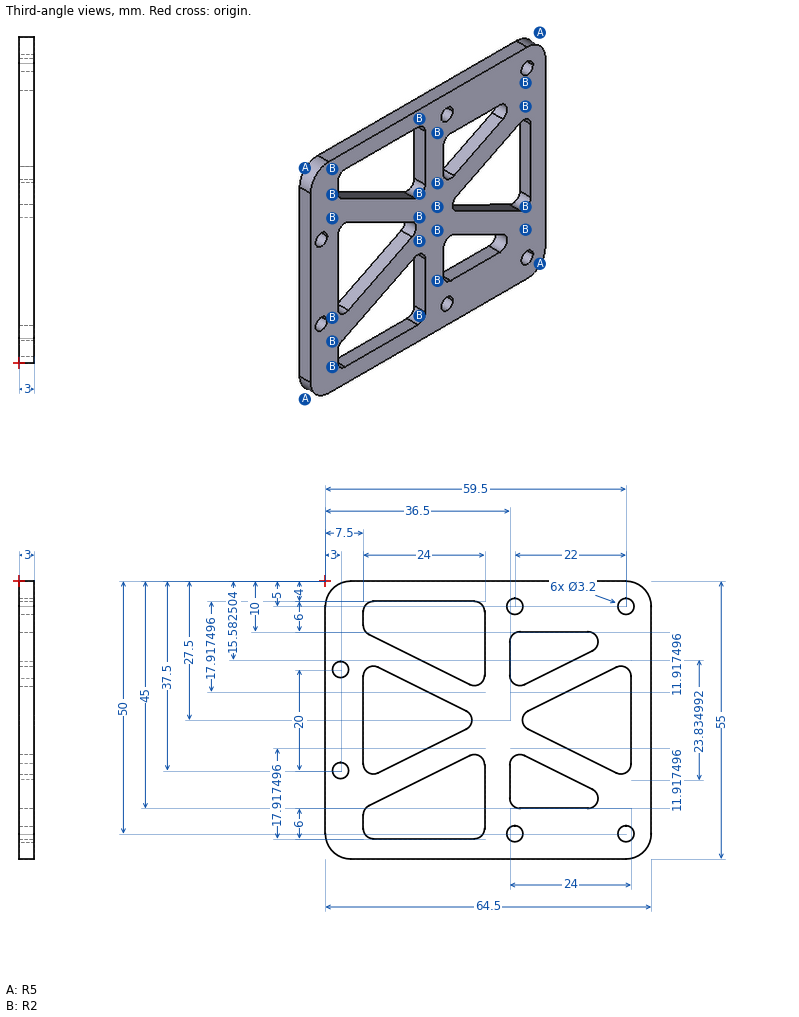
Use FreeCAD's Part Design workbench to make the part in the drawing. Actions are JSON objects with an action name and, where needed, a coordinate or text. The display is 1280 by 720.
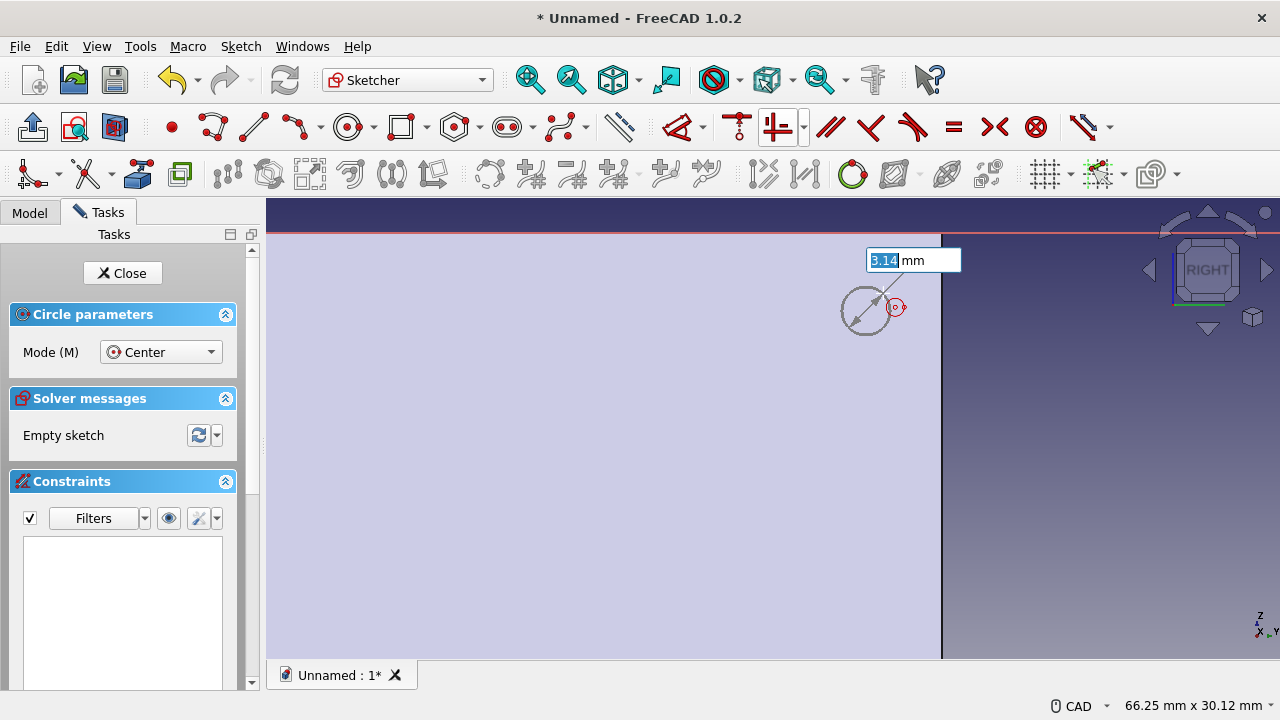
{"action": "type", "text": "3.2"}
{"action": "key", "text": "Return"}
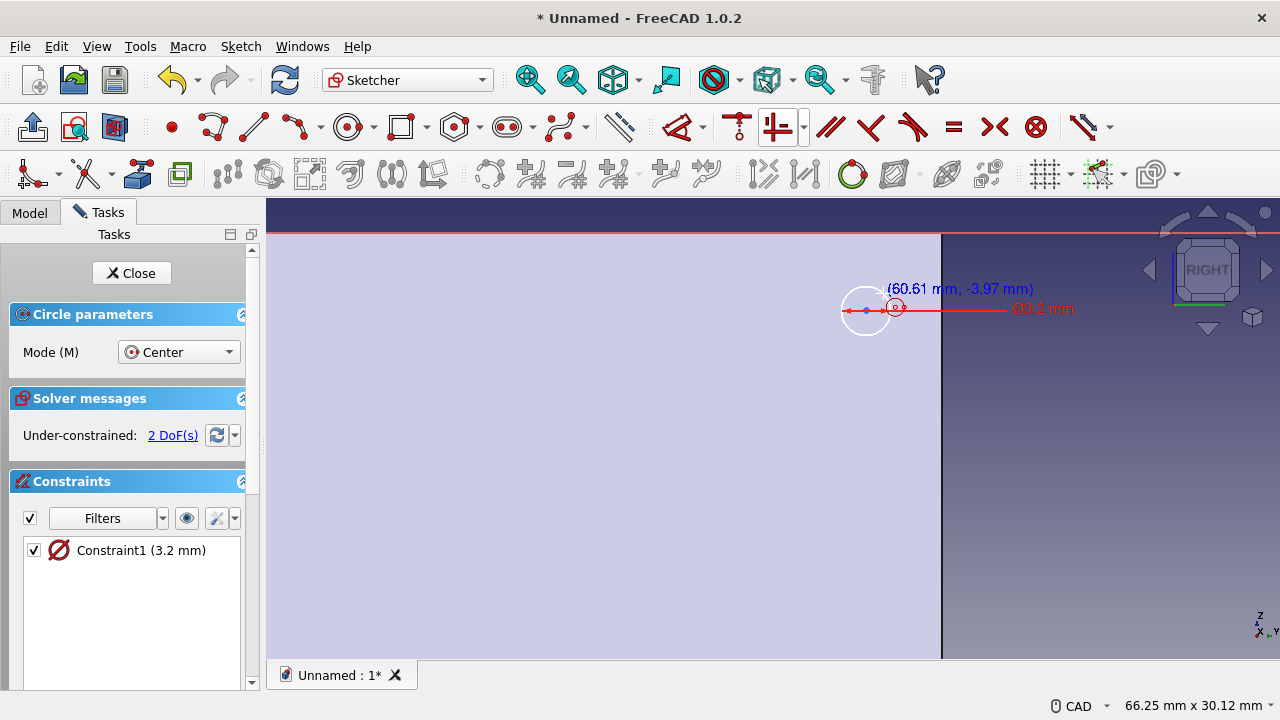
{"action": "left_click", "coordinate": [529, 310]}
{"action": "mouse_move", "coordinate": [547, 293]}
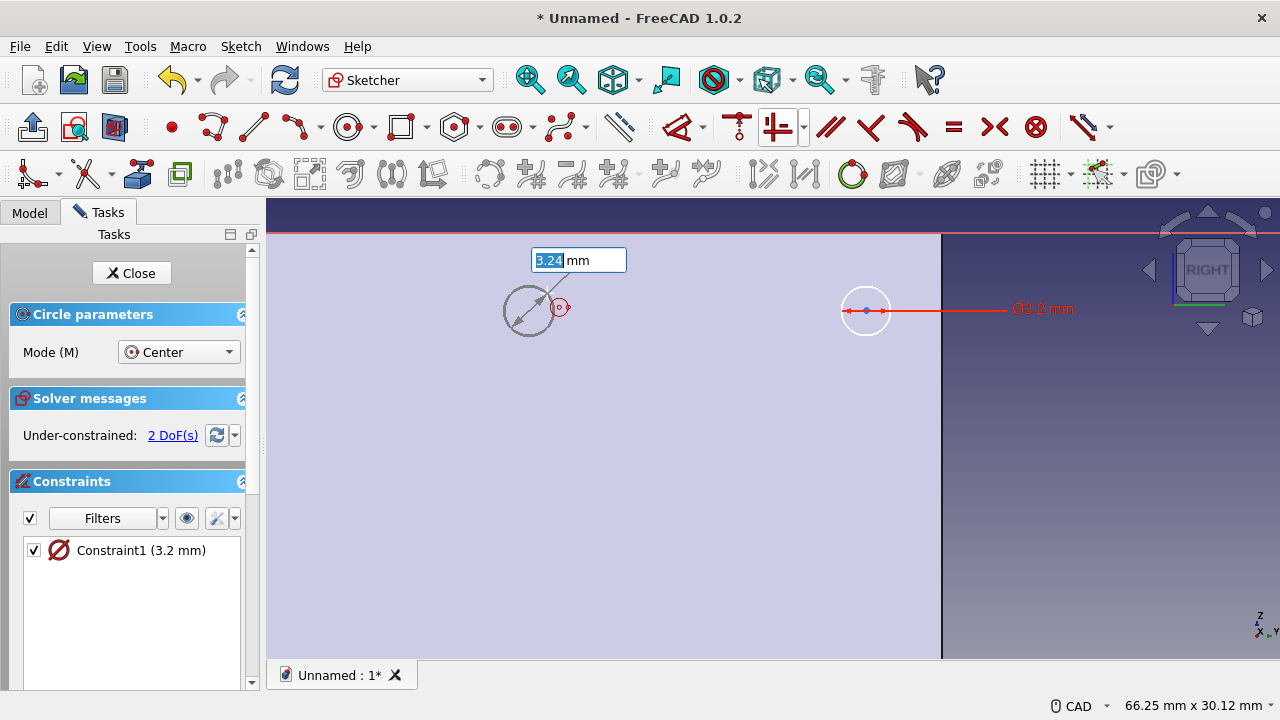
{"action": "type", "text": "3.2"}
{"action": "key", "text": "Return"}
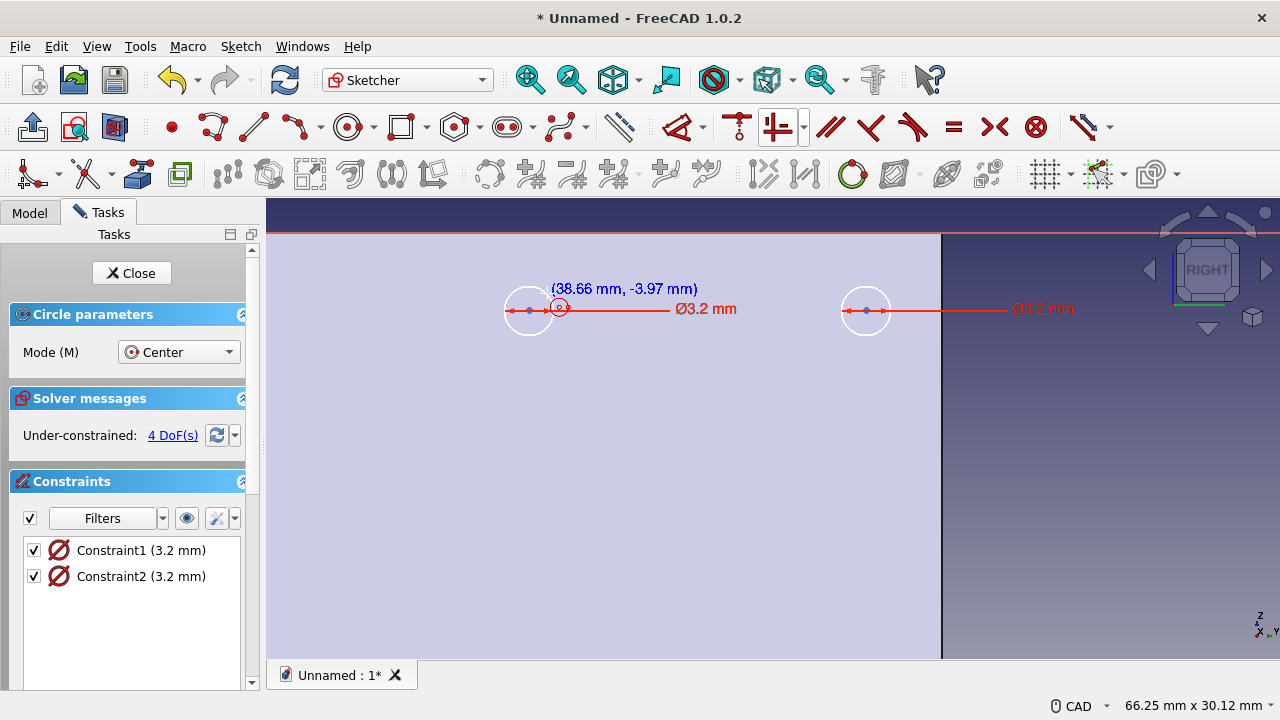
{"action": "scroll", "coordinate": [868, 312], "scroll_direction": "down", "scroll_amount": 5}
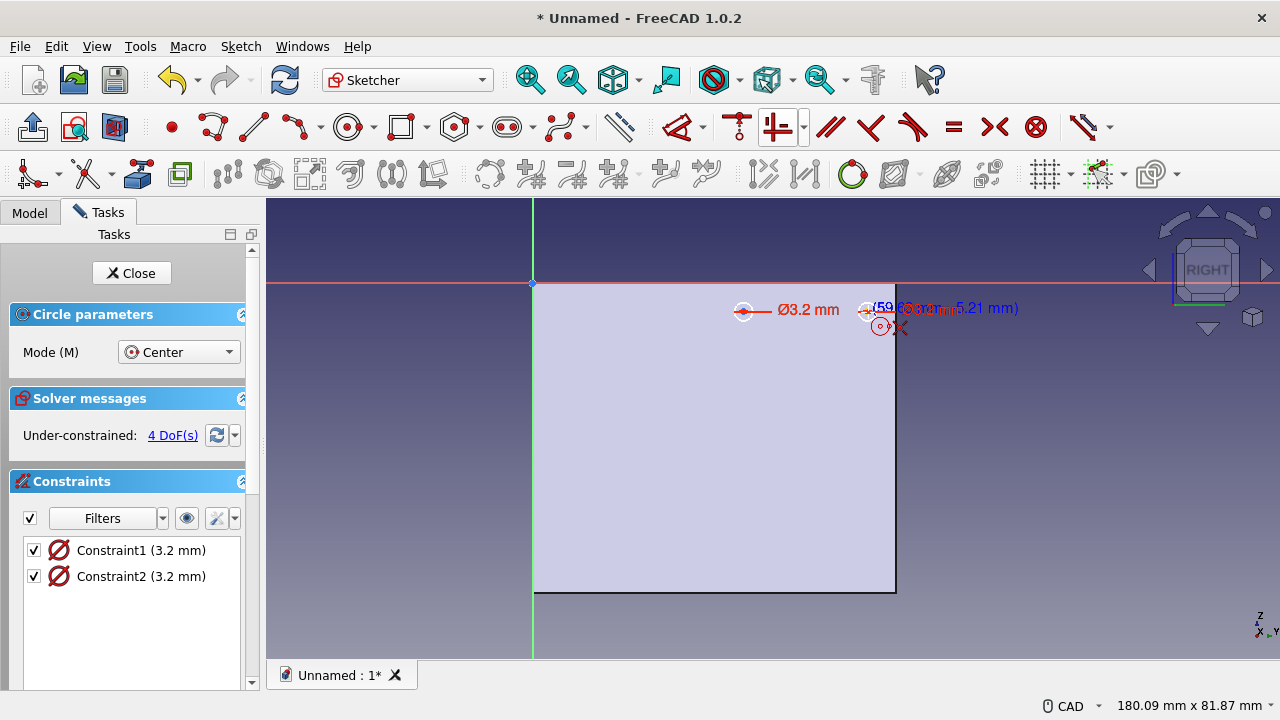
{"action": "scroll", "coordinate": [868, 565], "scroll_direction": "up", "scroll_amount": 5}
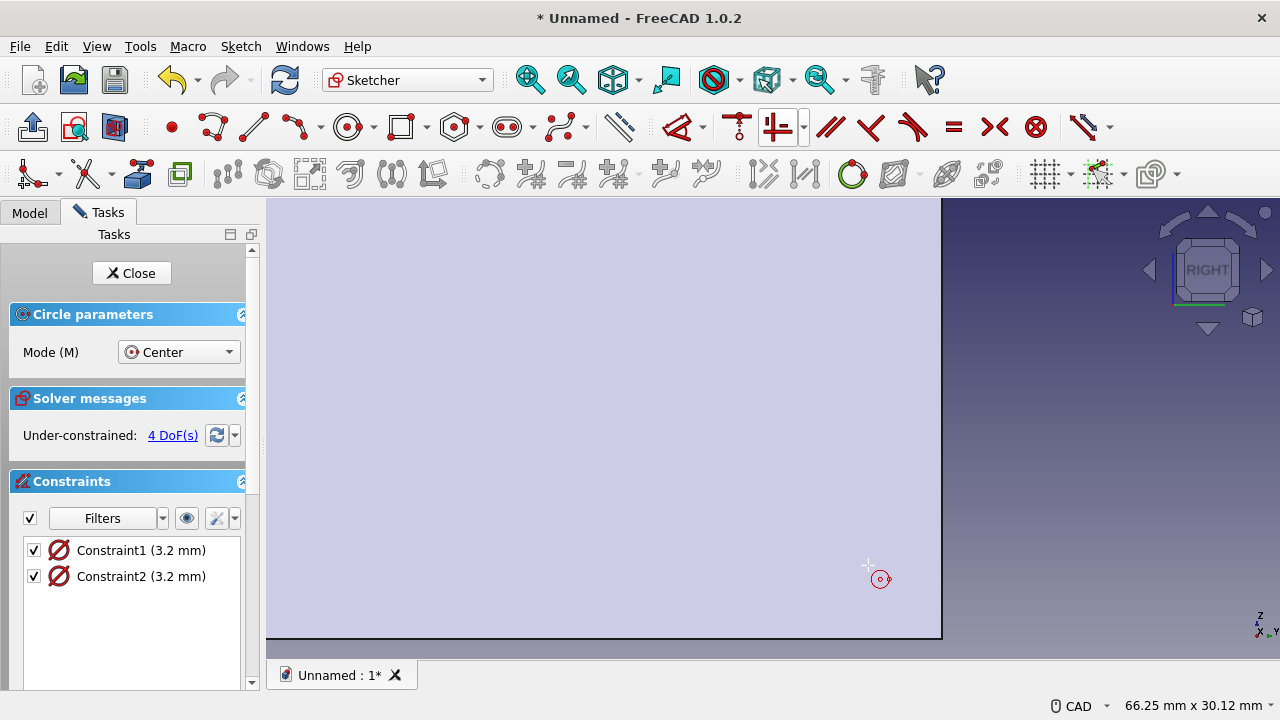
{"action": "left_click", "coordinate": [866, 563]}
{"action": "mouse_move", "coordinate": [883, 546]}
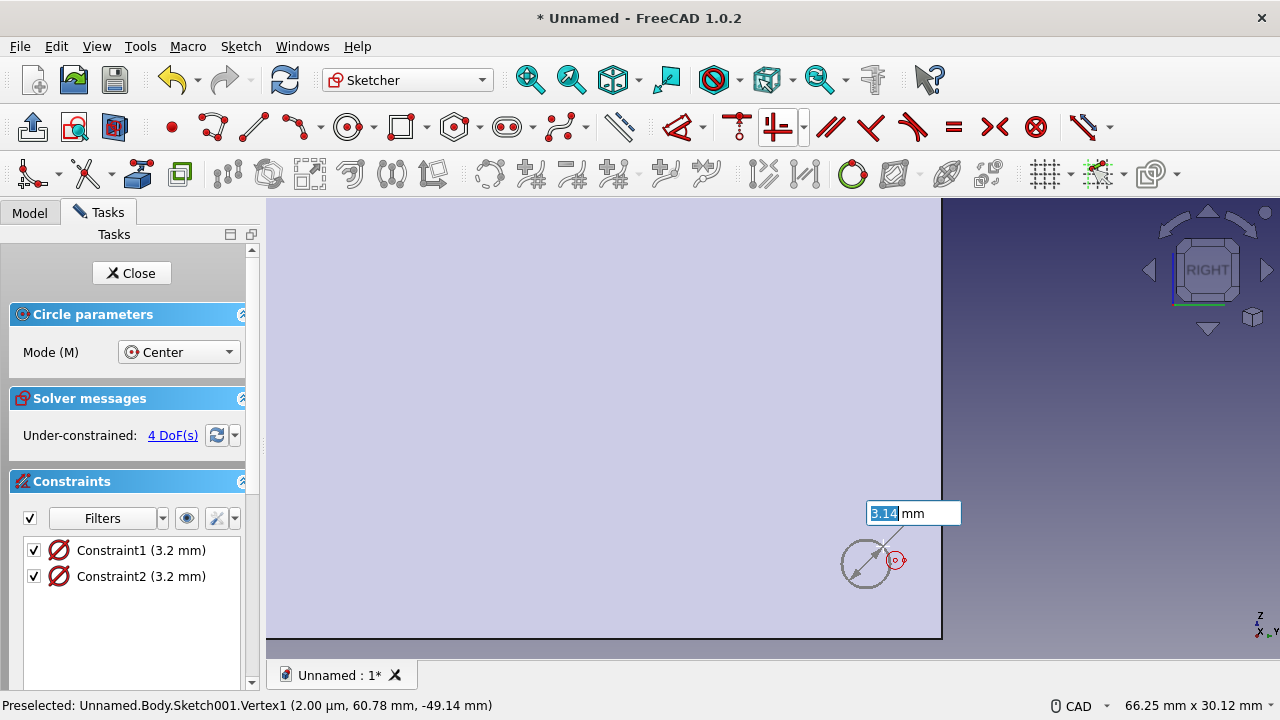
{"action": "type", "text": "3.2"}
{"action": "key", "text": "Return"}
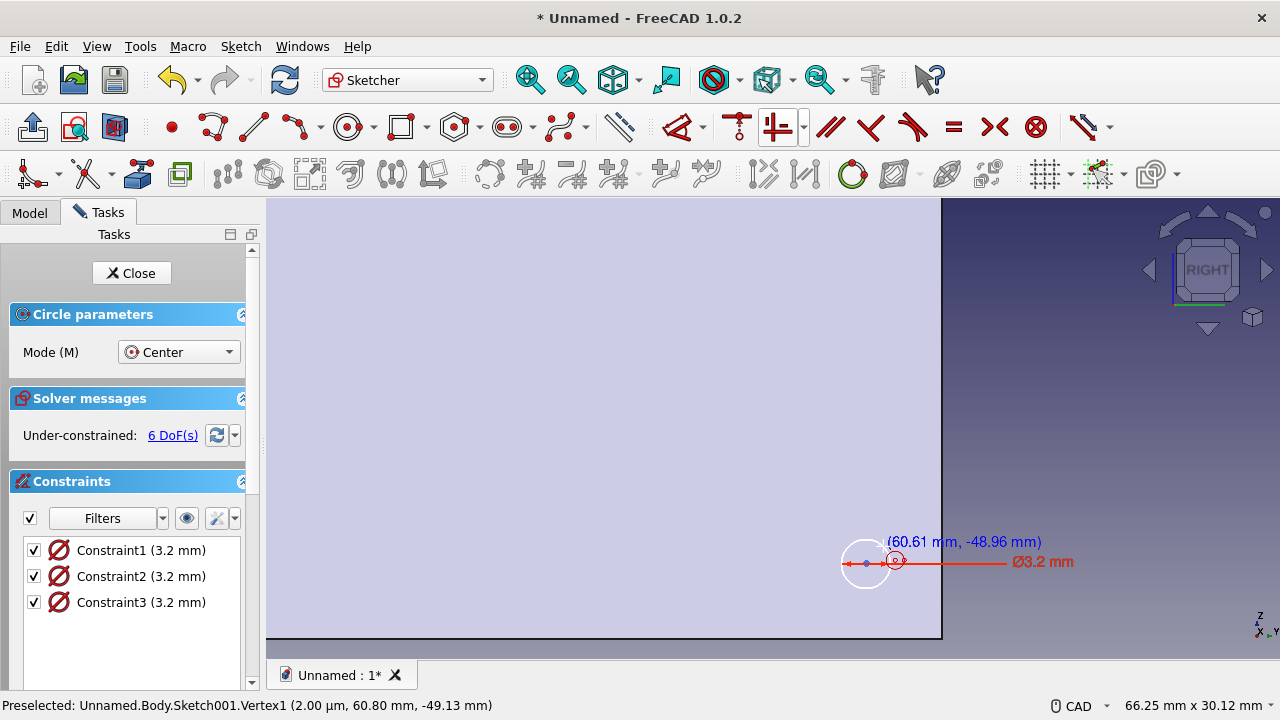
{"action": "left_click", "coordinate": [529, 563]}
{"action": "mouse_move", "coordinate": [547, 546]}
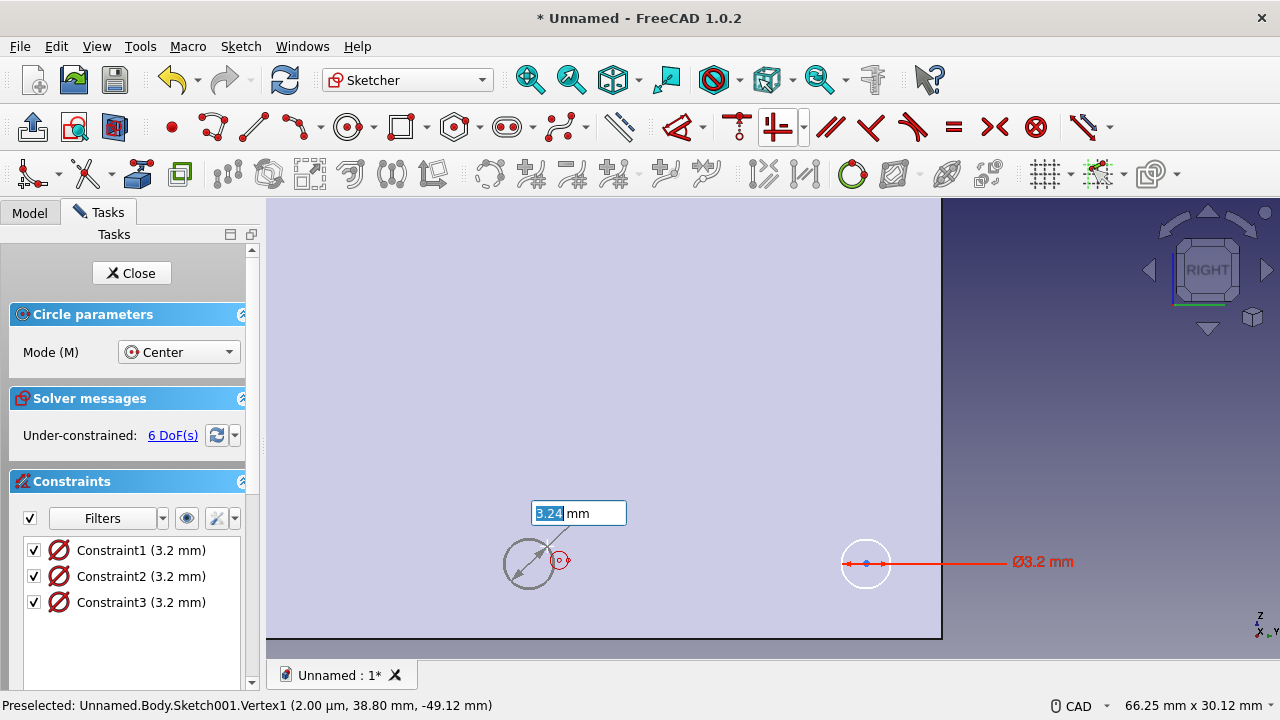
{"action": "type", "text": "3.2"}
{"action": "key", "text": "Return"}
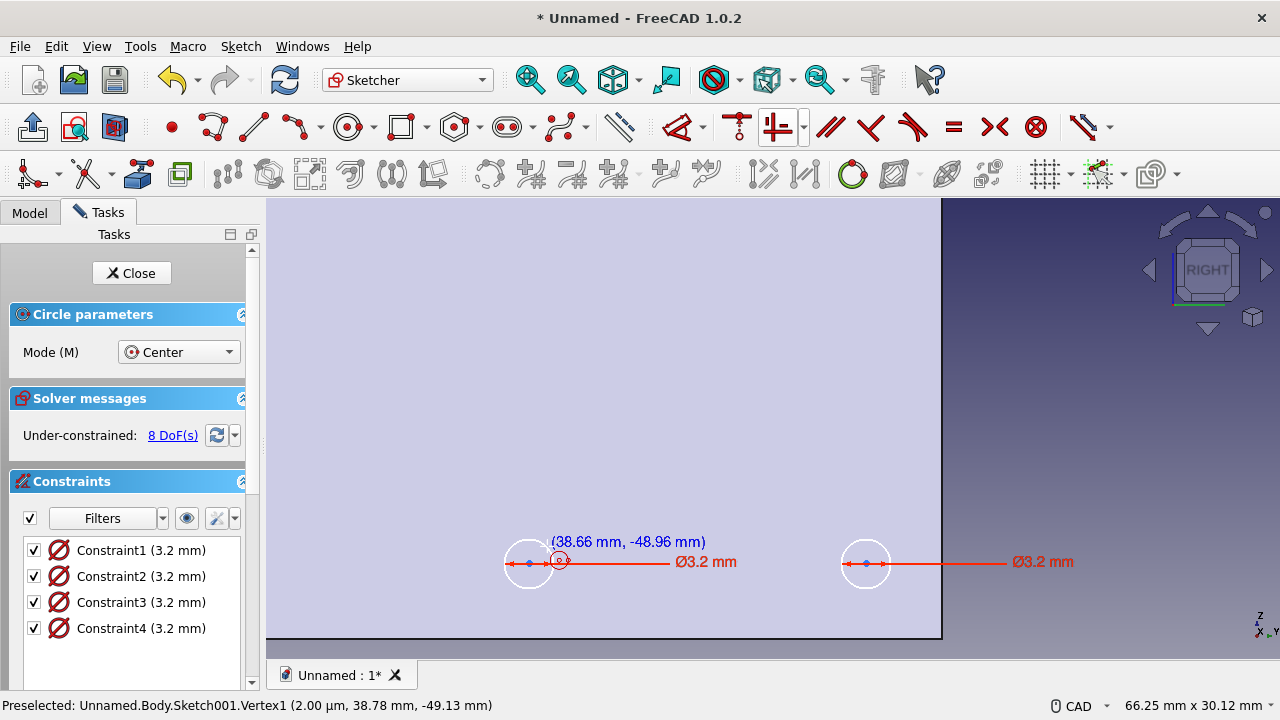
{"action": "scroll", "coordinate": [868, 566], "scroll_direction": "down", "scroll_amount": 5}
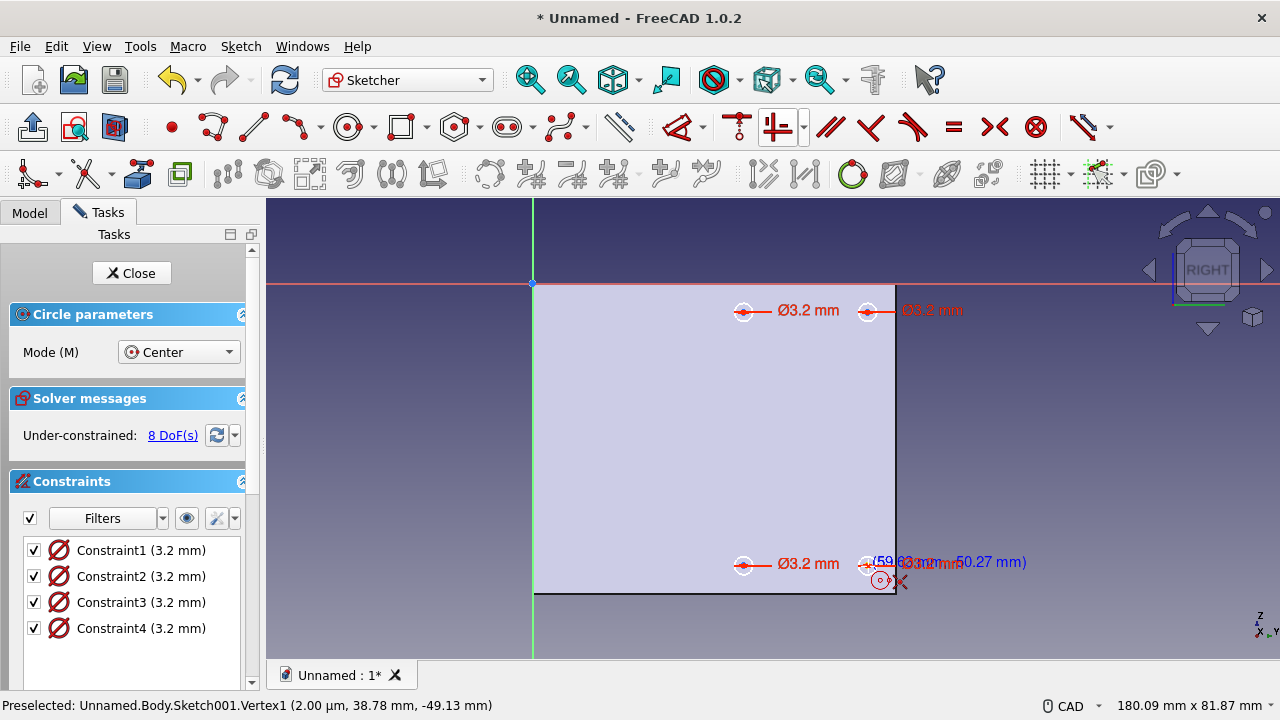
{"action": "scroll", "coordinate": [549, 495], "scroll_direction": "up", "scroll_amount": 5}